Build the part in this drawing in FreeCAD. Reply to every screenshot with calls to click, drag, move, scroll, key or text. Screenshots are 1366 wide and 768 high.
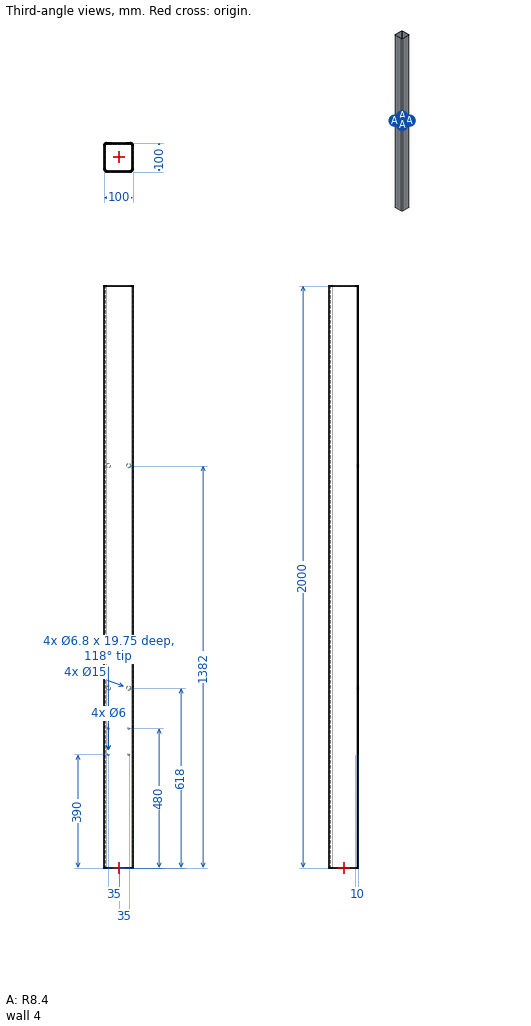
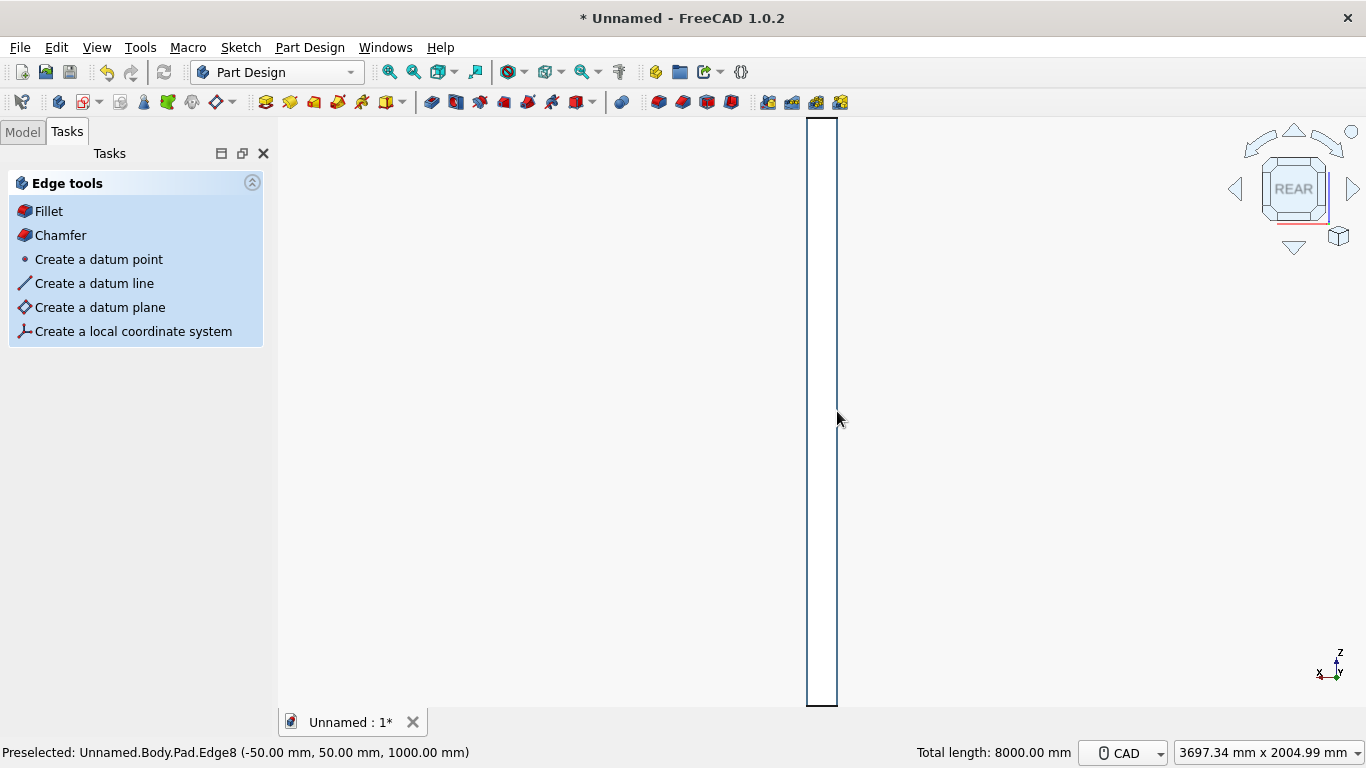
click(660, 102)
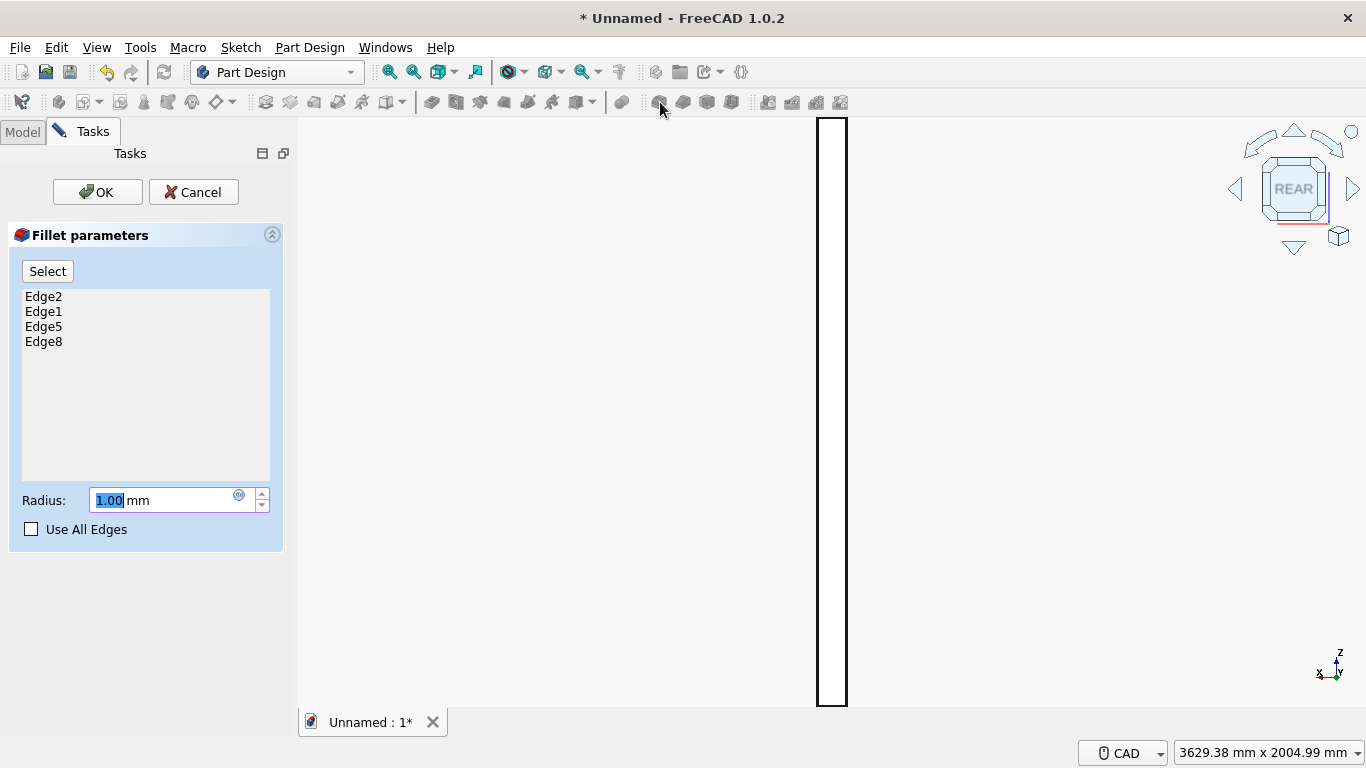
text(8.4)
key(Tab)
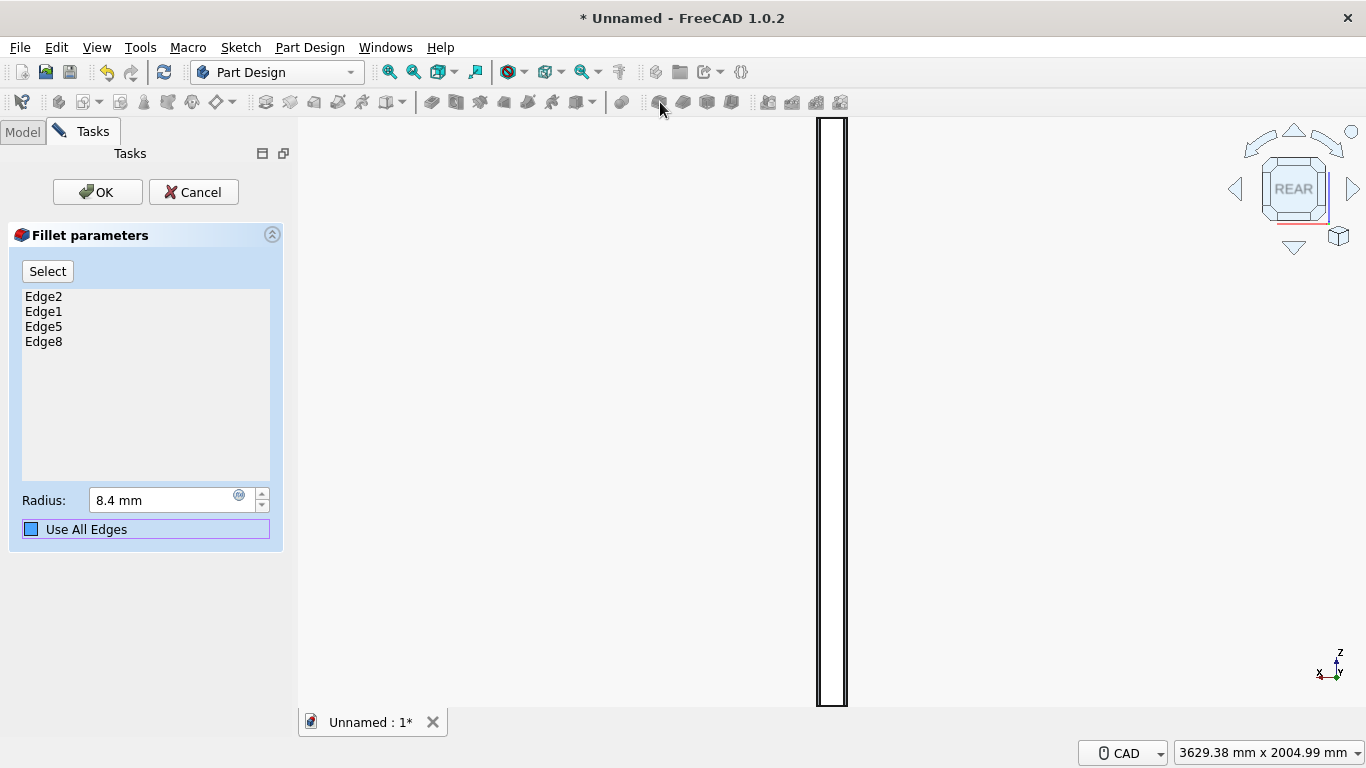
click(98, 192)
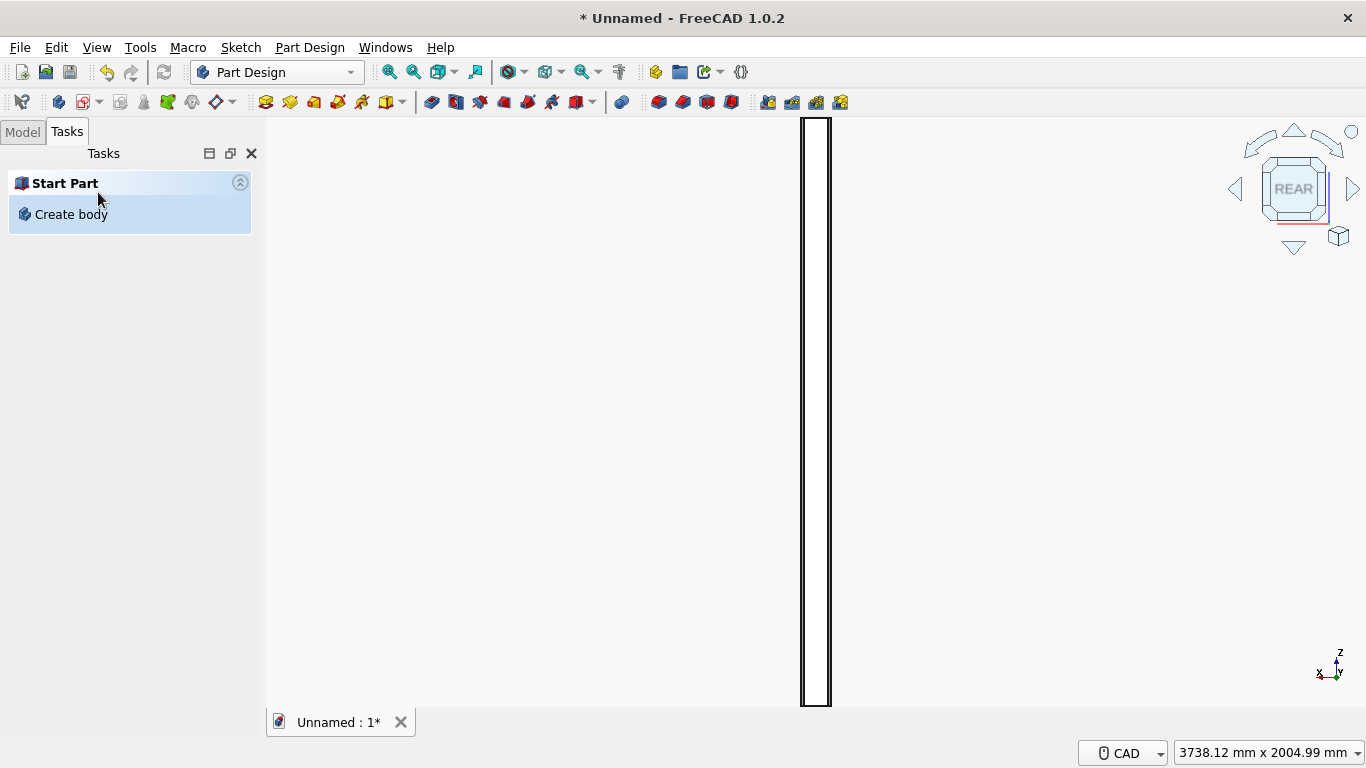
key(0)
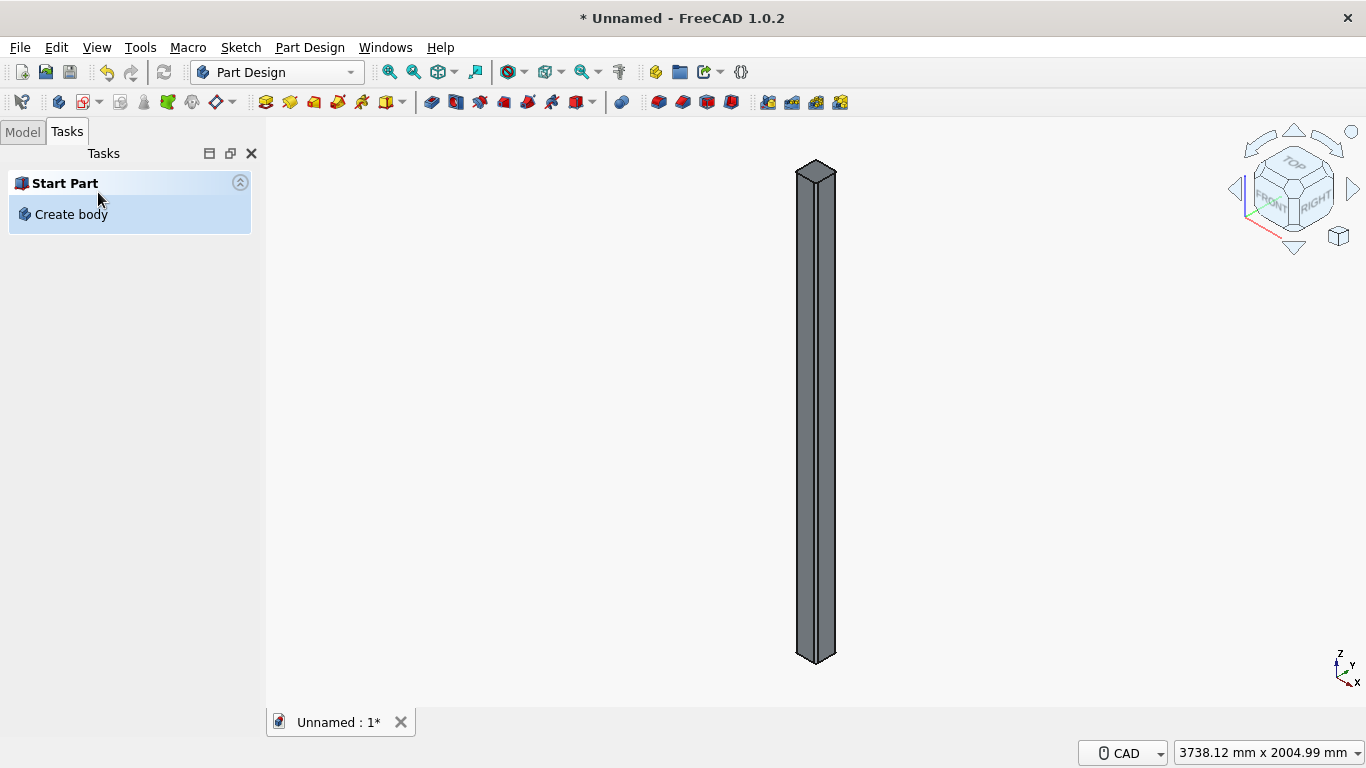
click(816, 171)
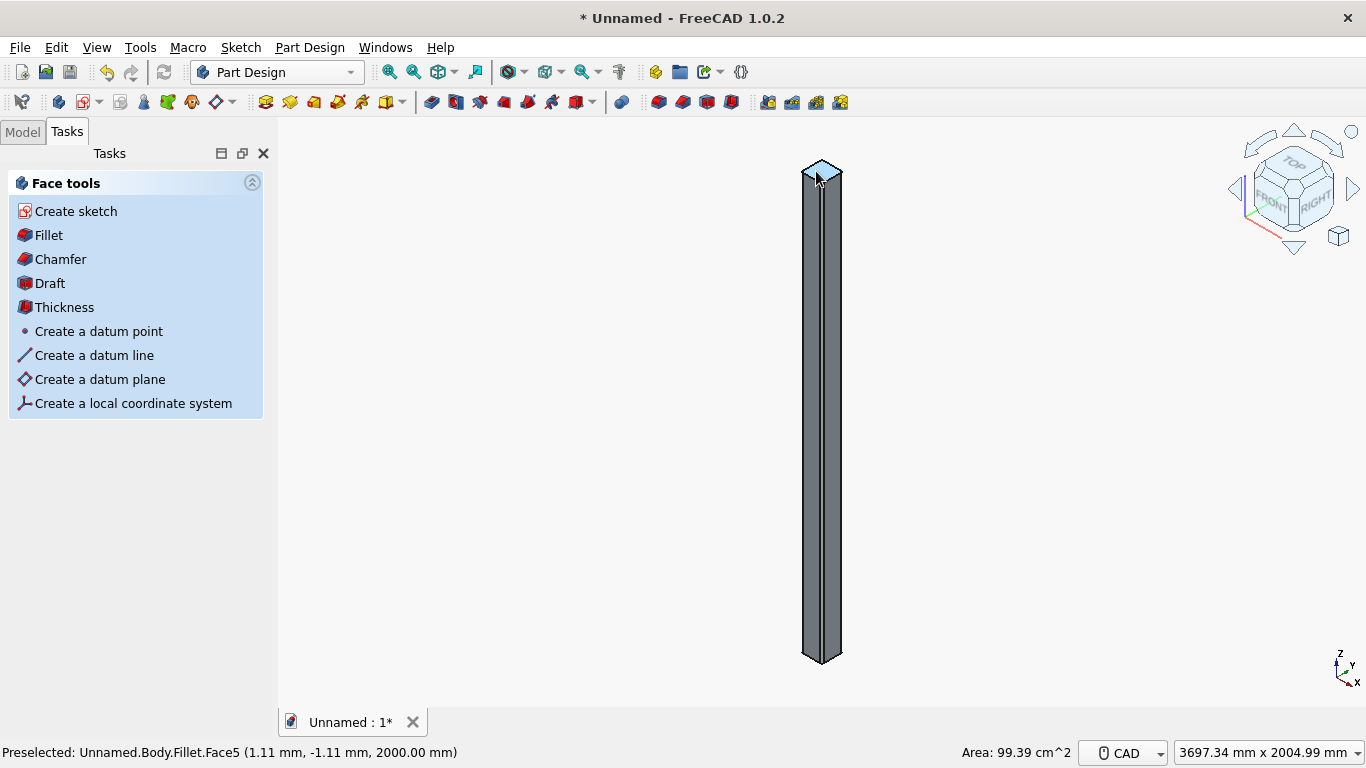
key(2)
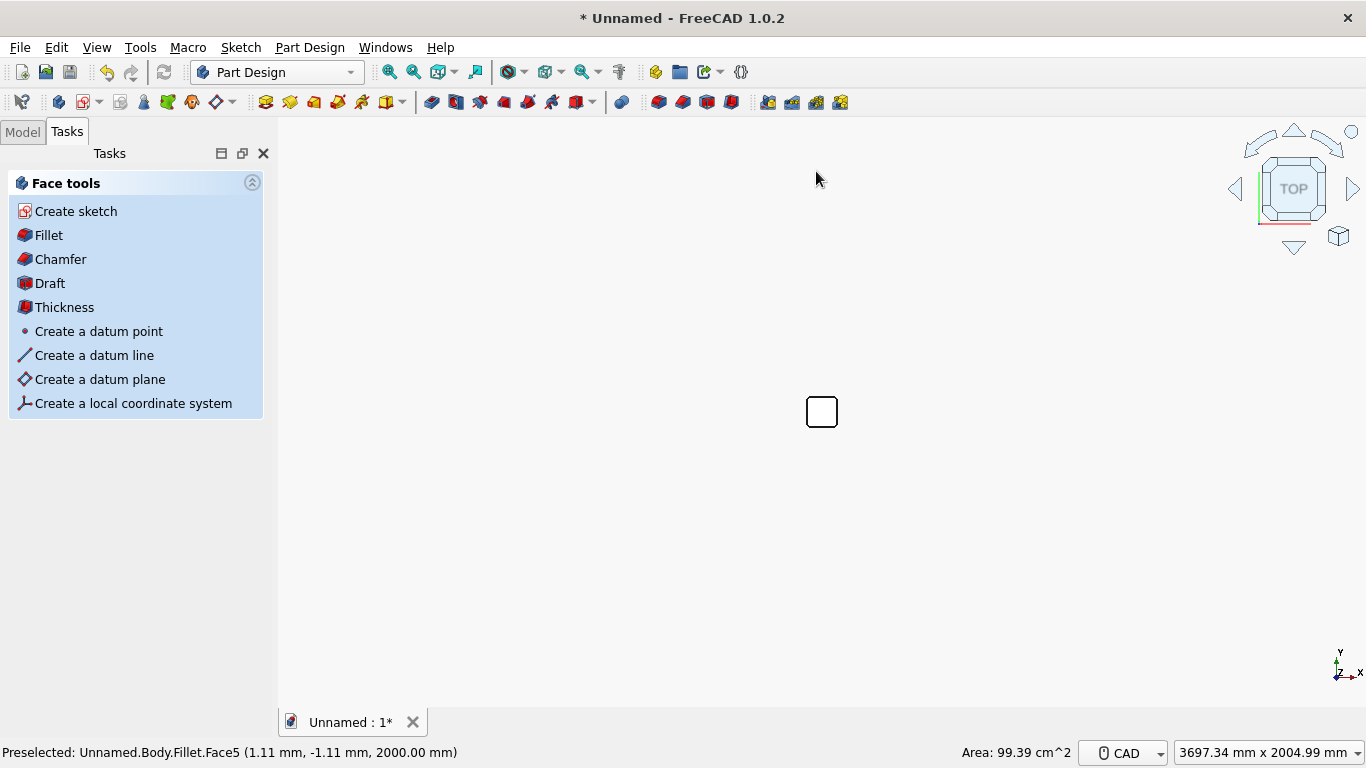
click(390, 72)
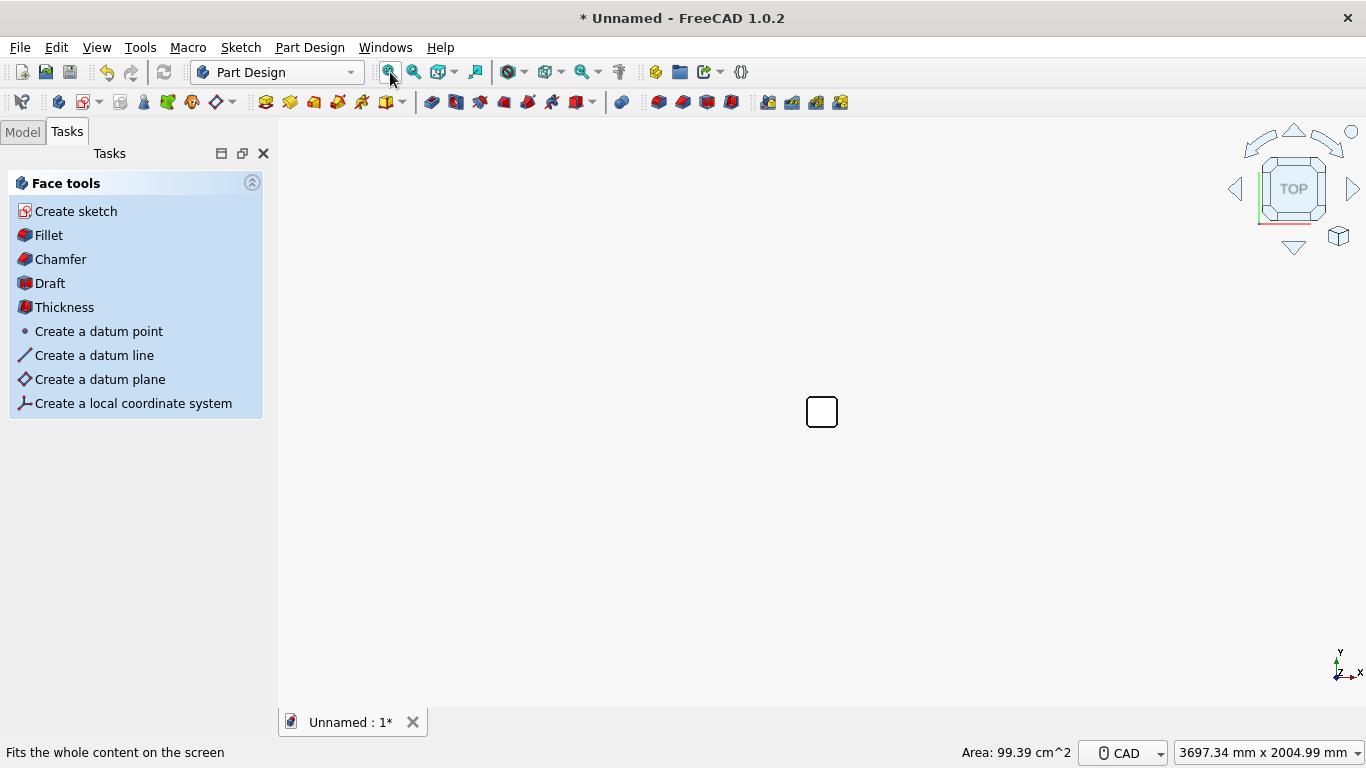
key(1)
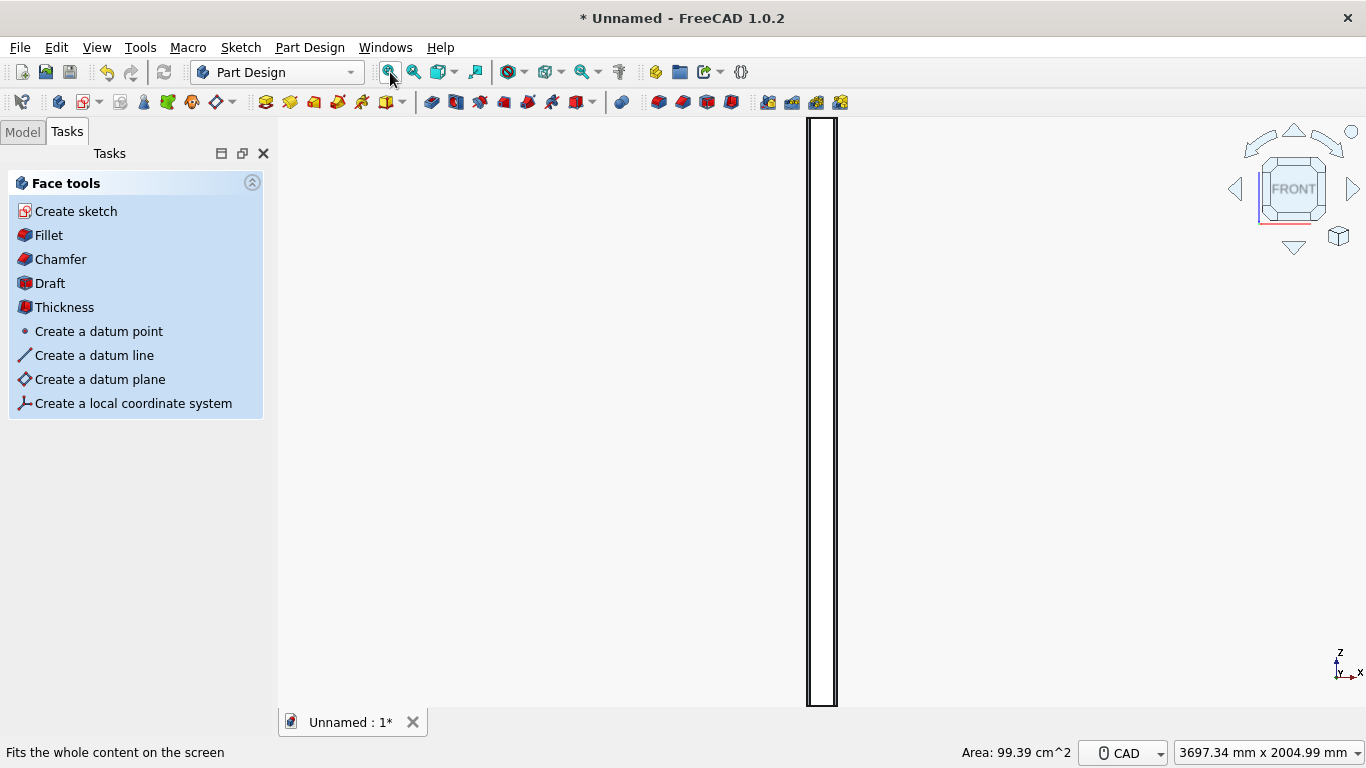
key(3)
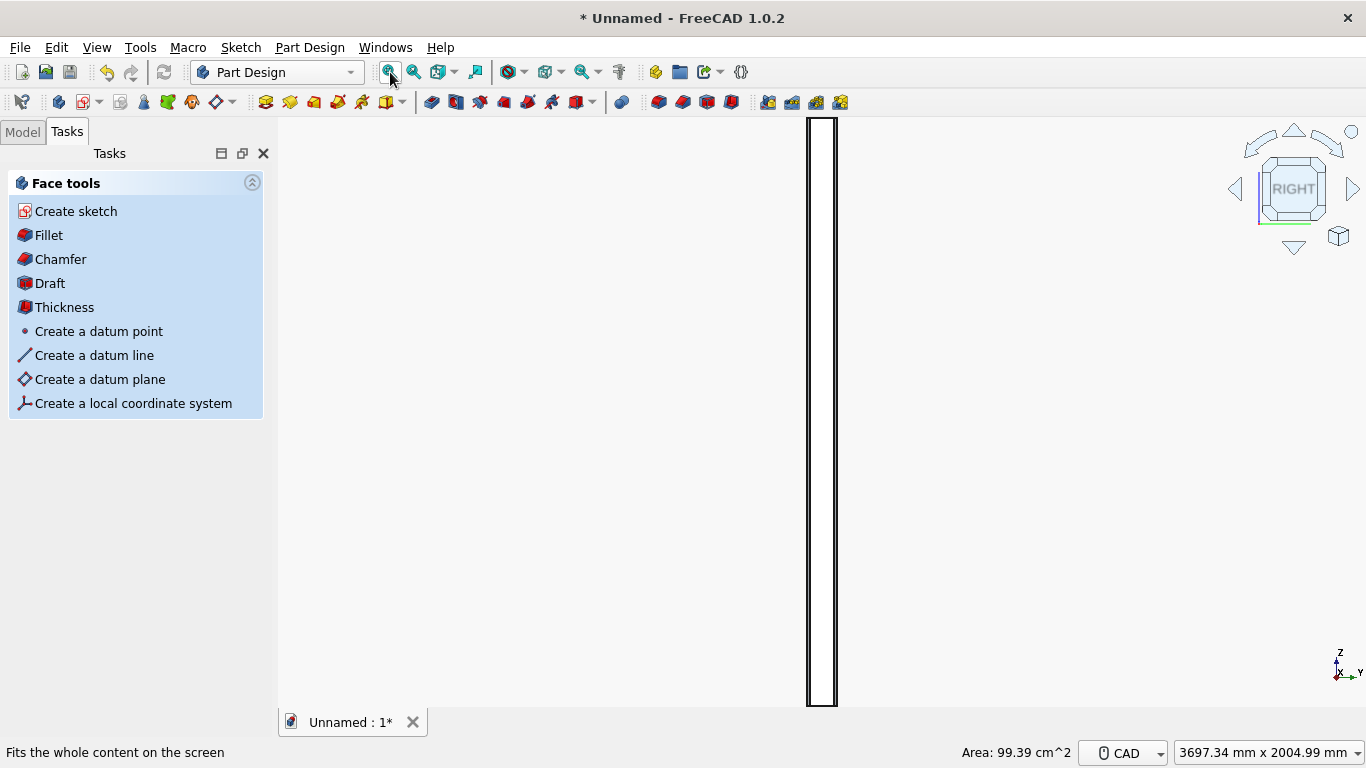
key(5)